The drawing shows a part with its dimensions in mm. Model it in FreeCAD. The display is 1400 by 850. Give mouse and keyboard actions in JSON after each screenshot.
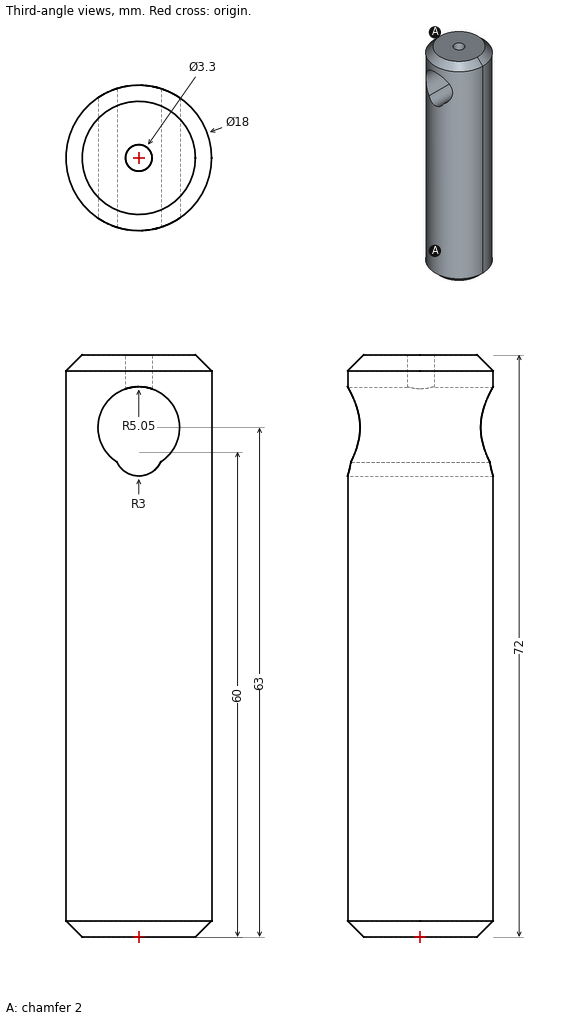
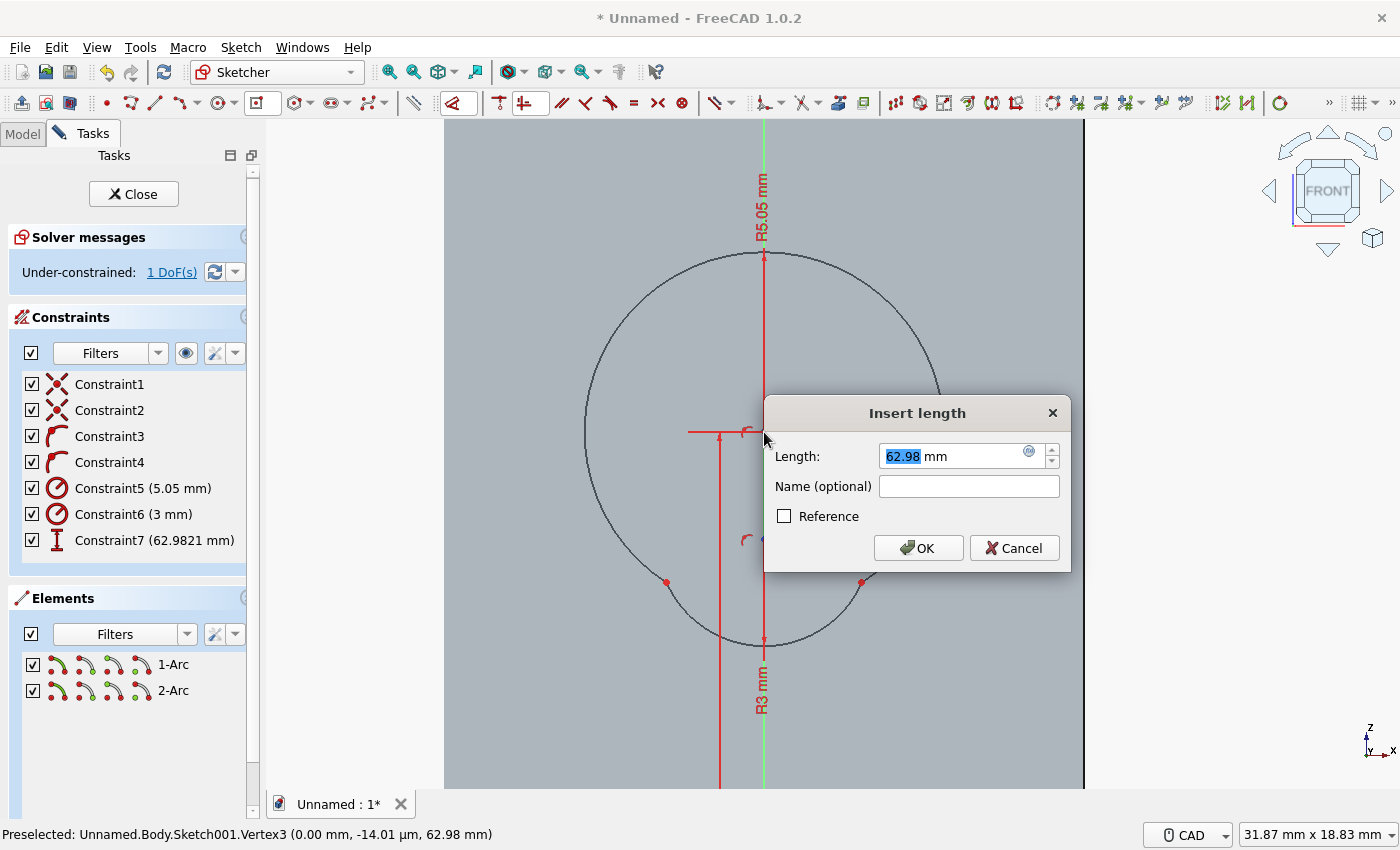
{"action": "type", "text": "63"}
{"action": "key", "text": "Return"}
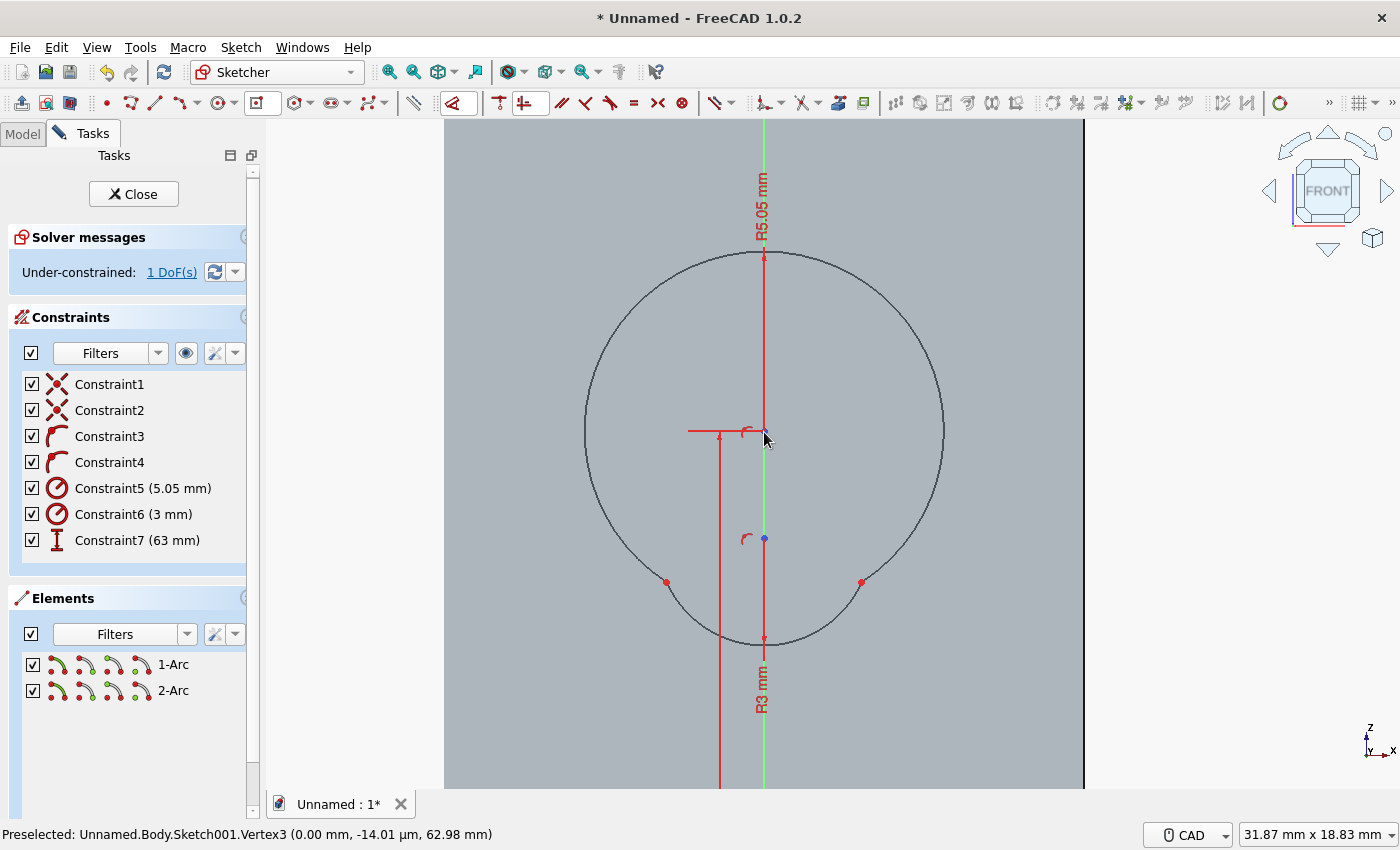
{"action": "left_click", "coordinate": [764, 539]}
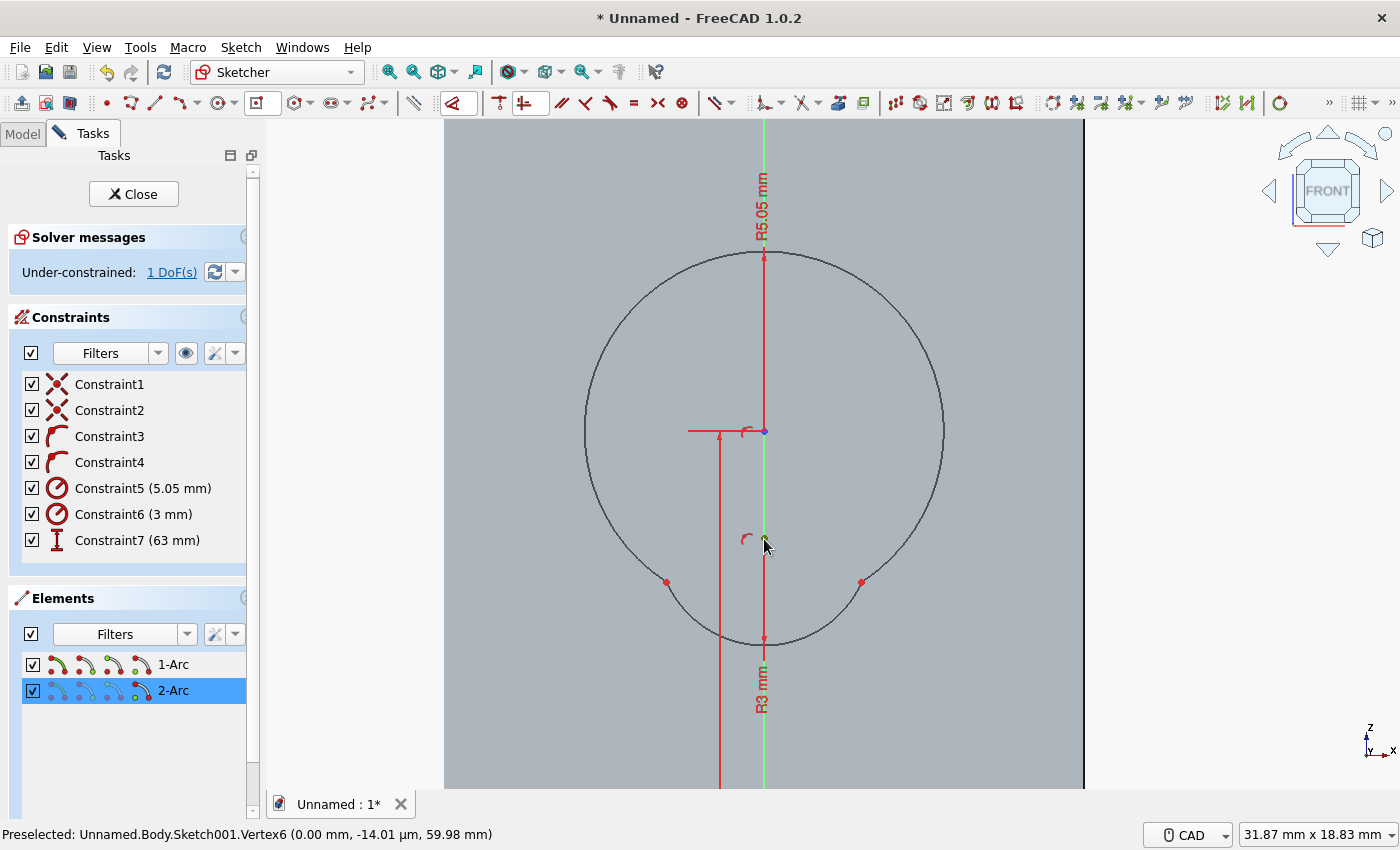
{"action": "left_click", "coordinate": [472, 104]}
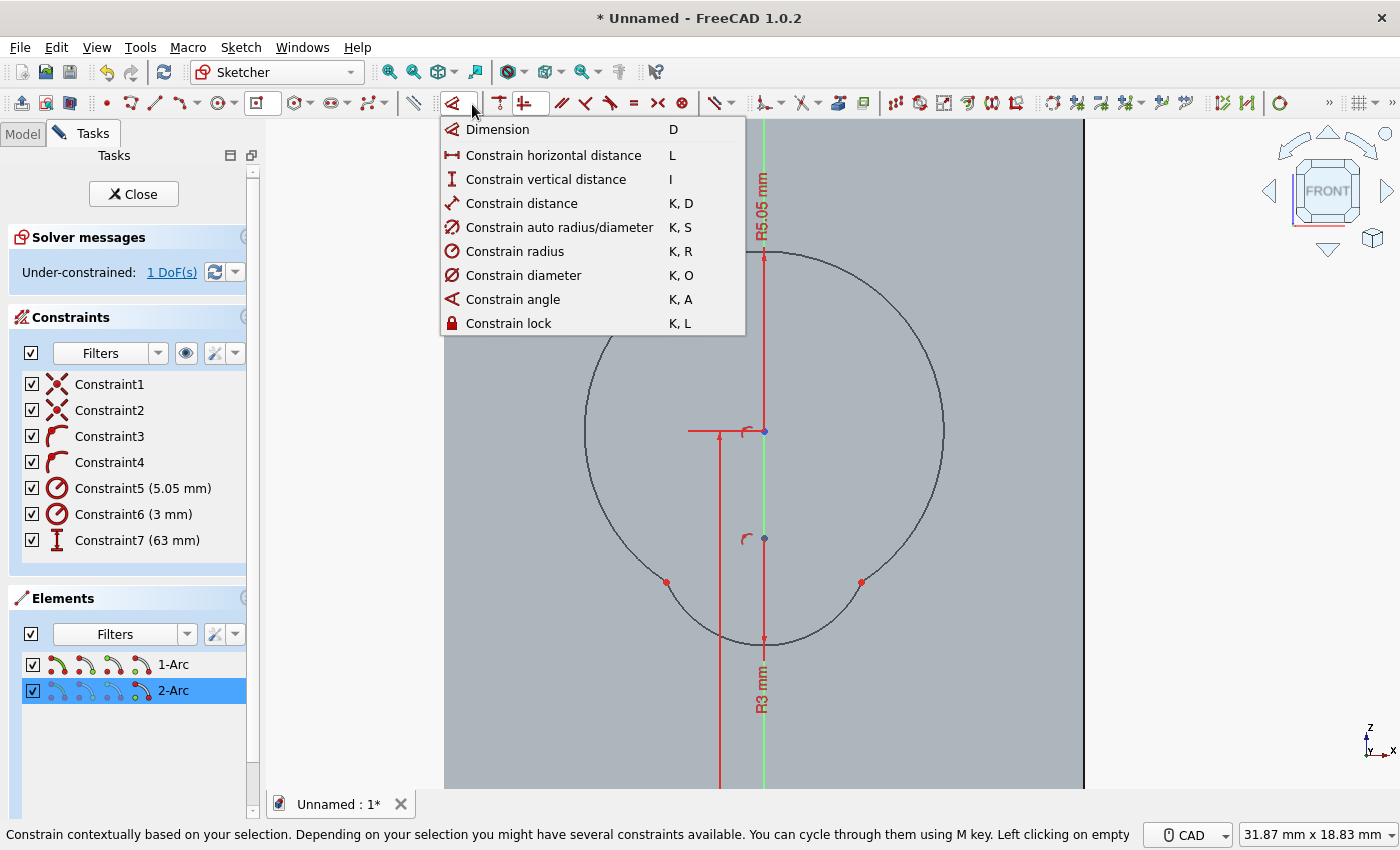
{"action": "left_click", "coordinate": [593, 179]}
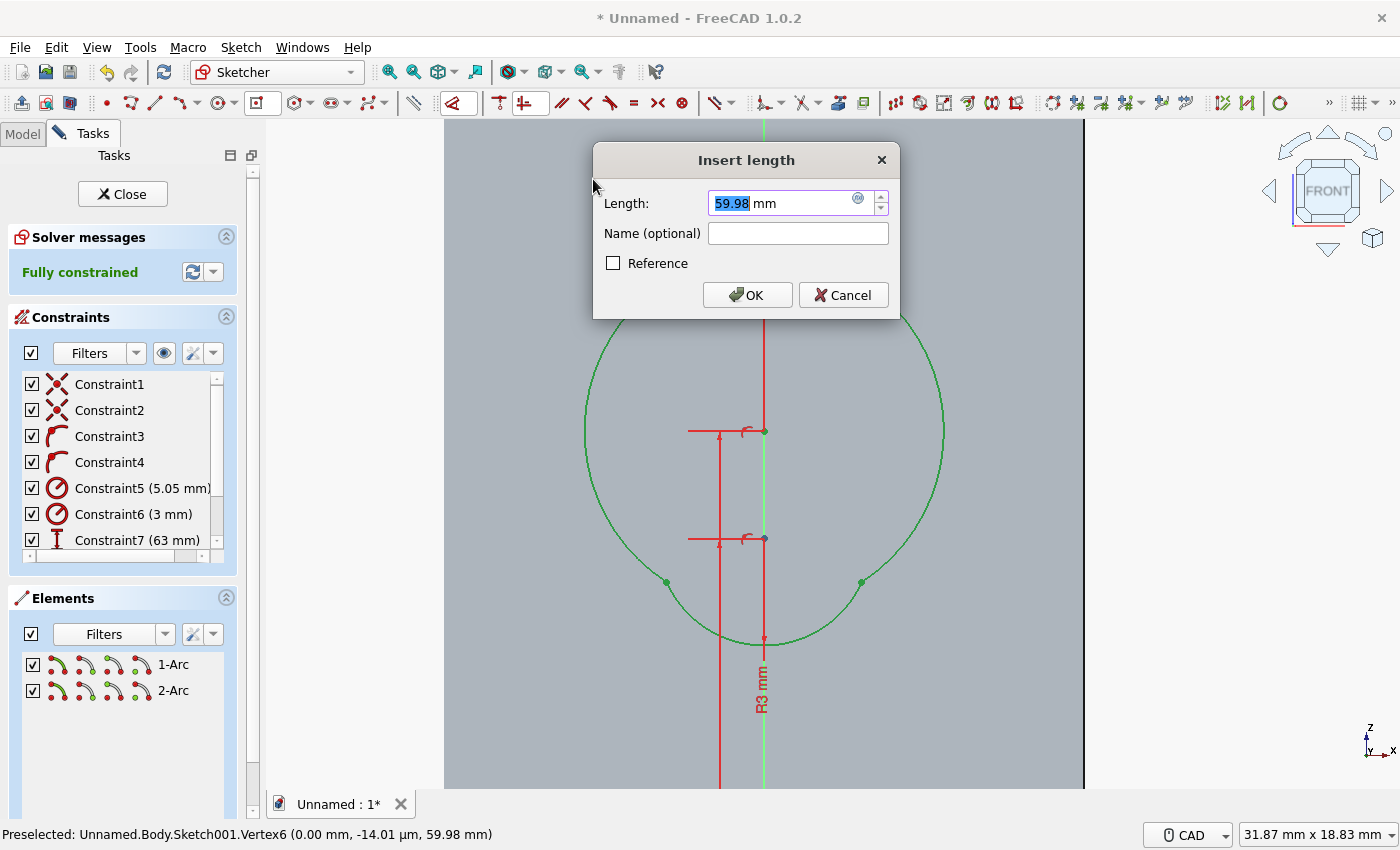
{"action": "type", "text": "60"}
{"action": "key", "text": "Return"}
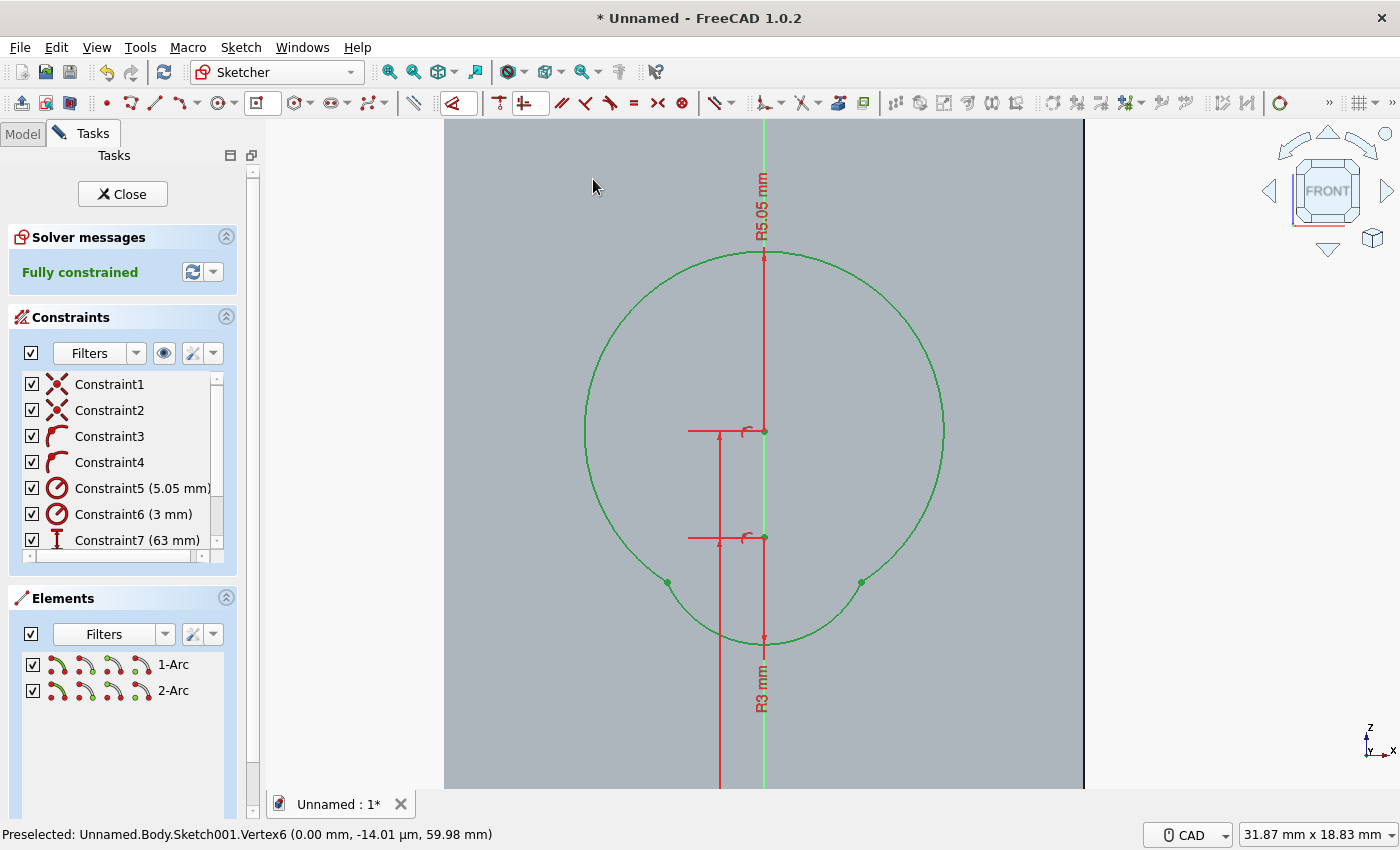
{"action": "left_click", "coordinate": [123, 194]}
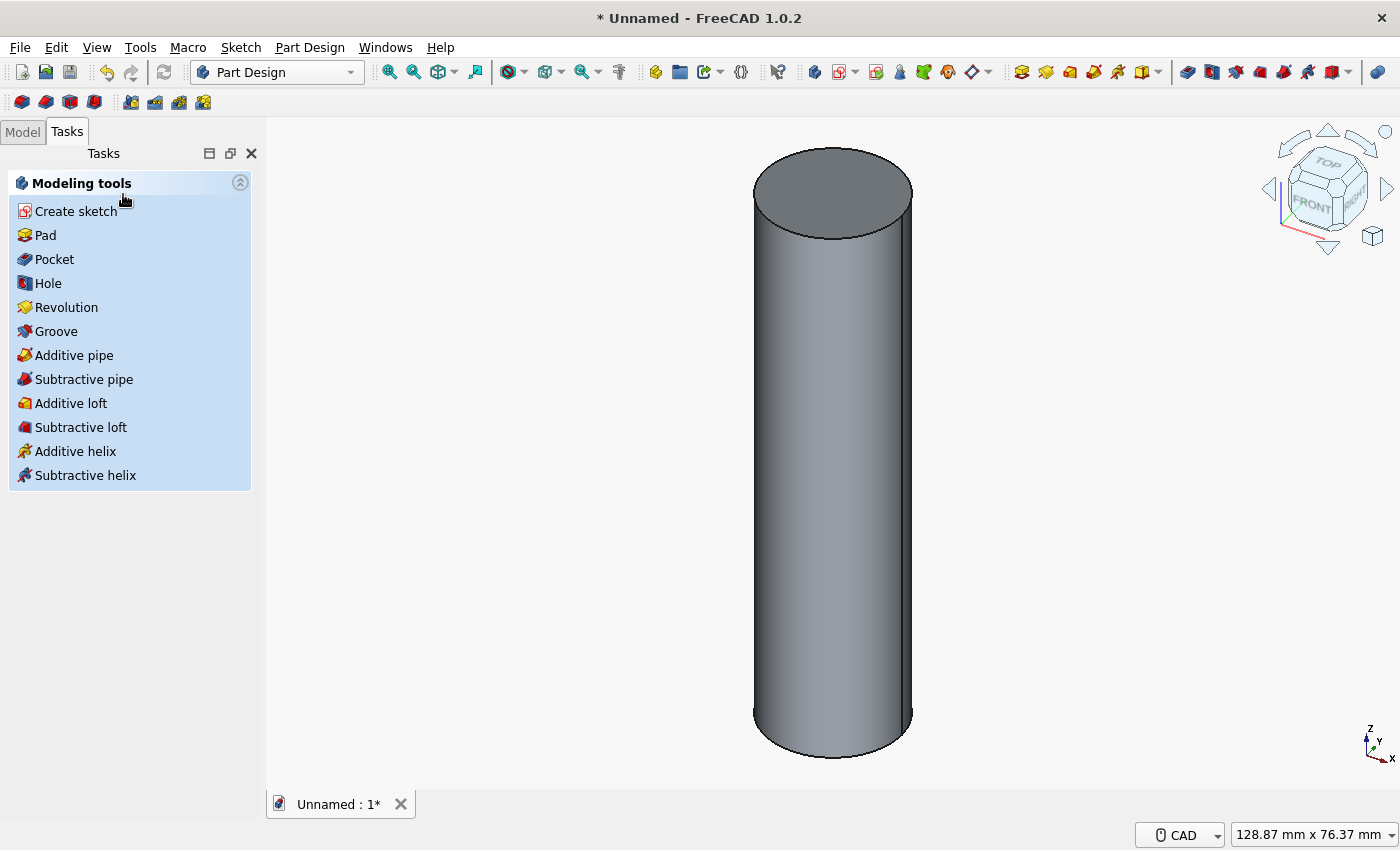
{"action": "left_click", "coordinate": [1188, 72]}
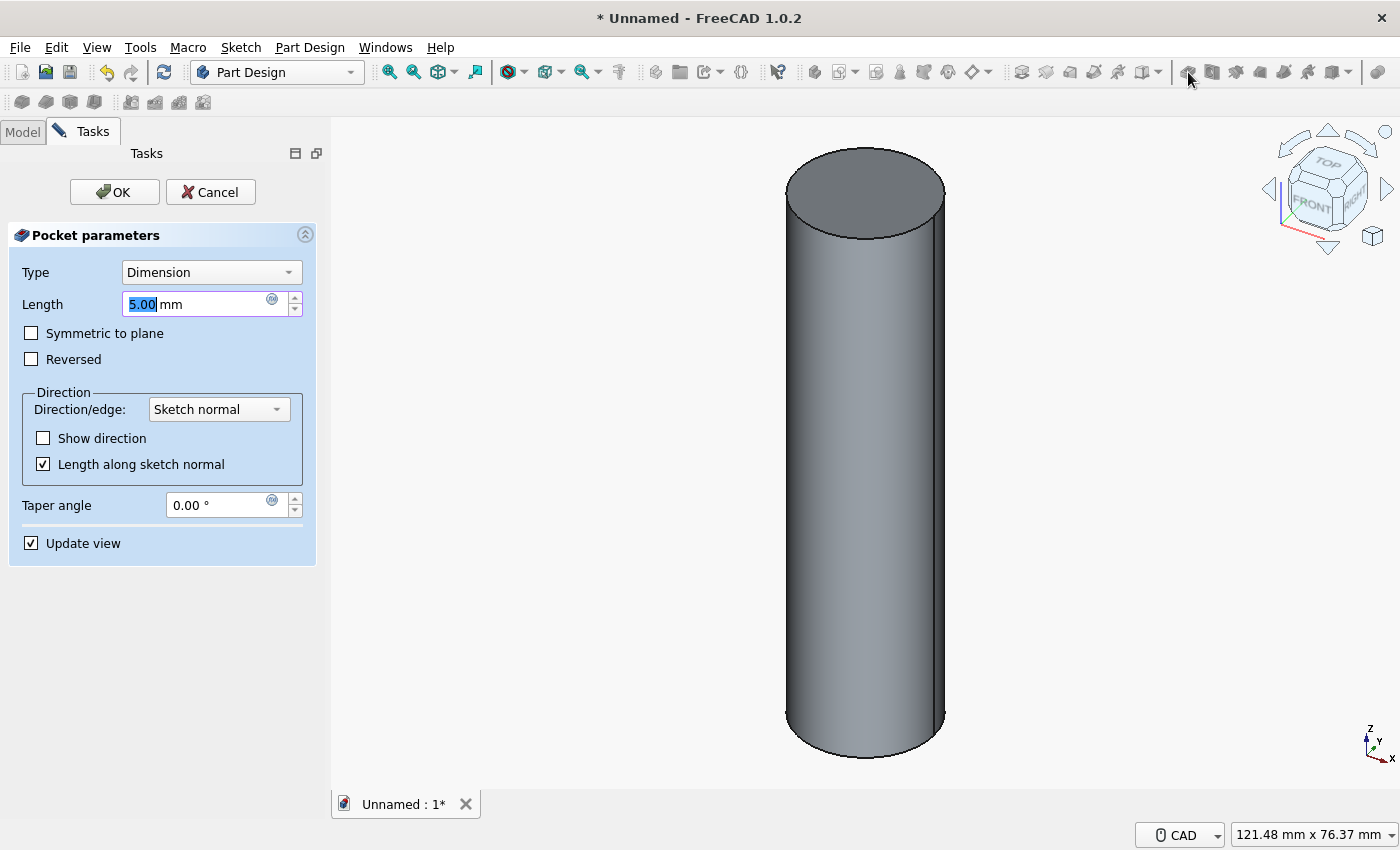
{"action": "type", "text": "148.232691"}
{"action": "key", "text": "Tab"}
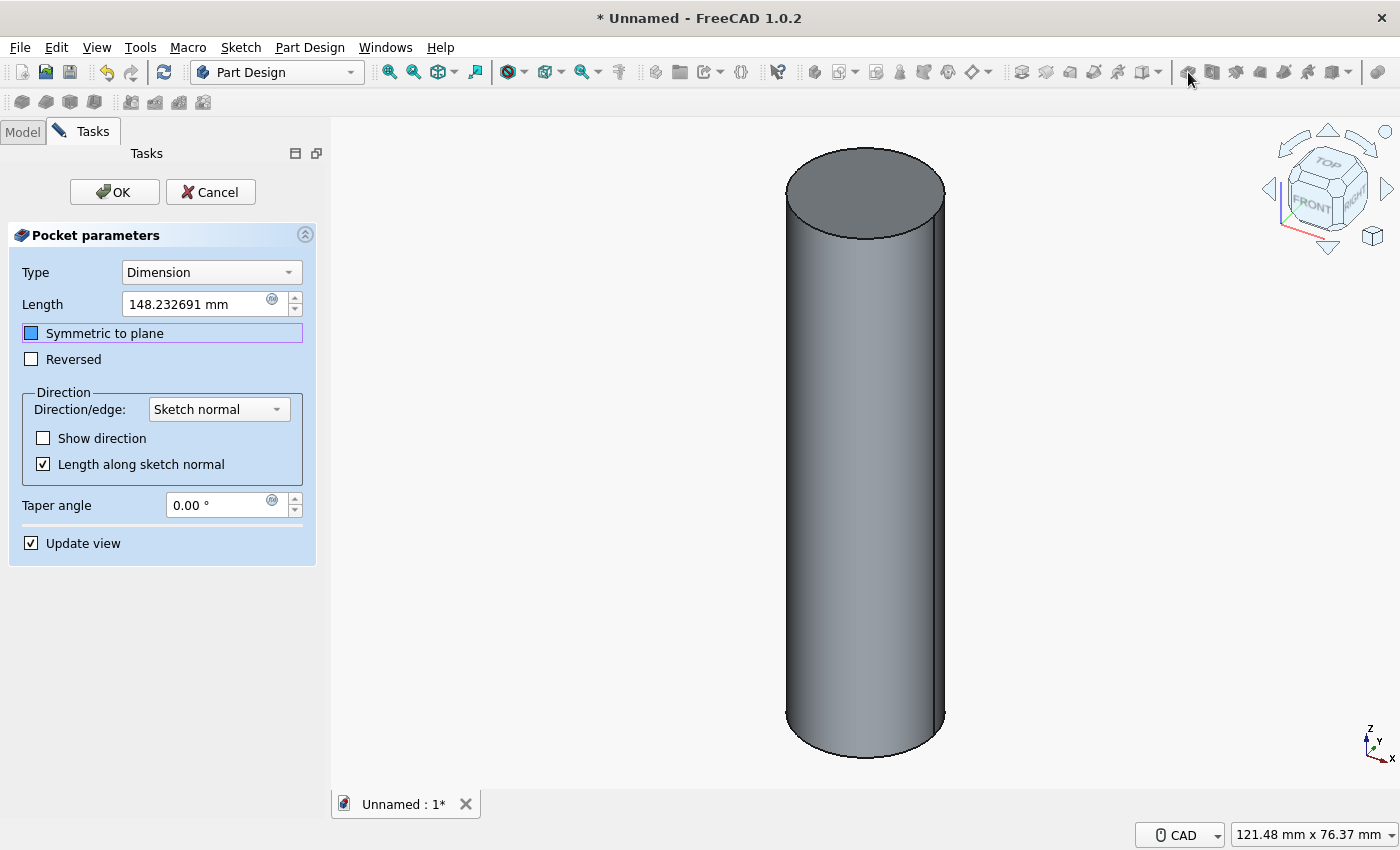
{"action": "left_click", "coordinate": [30, 333]}